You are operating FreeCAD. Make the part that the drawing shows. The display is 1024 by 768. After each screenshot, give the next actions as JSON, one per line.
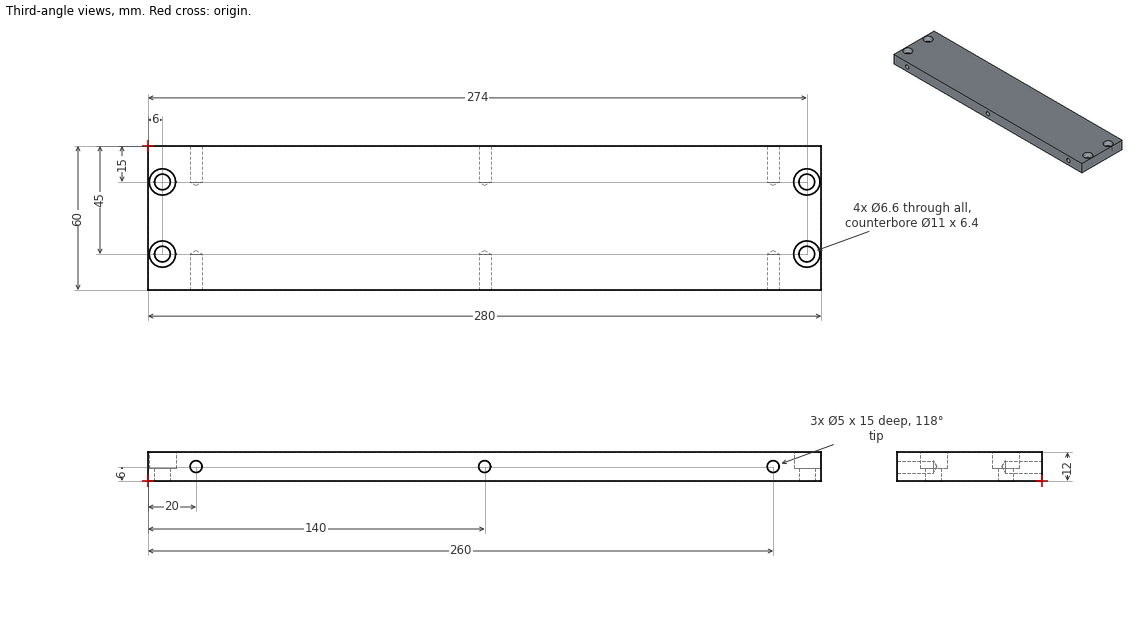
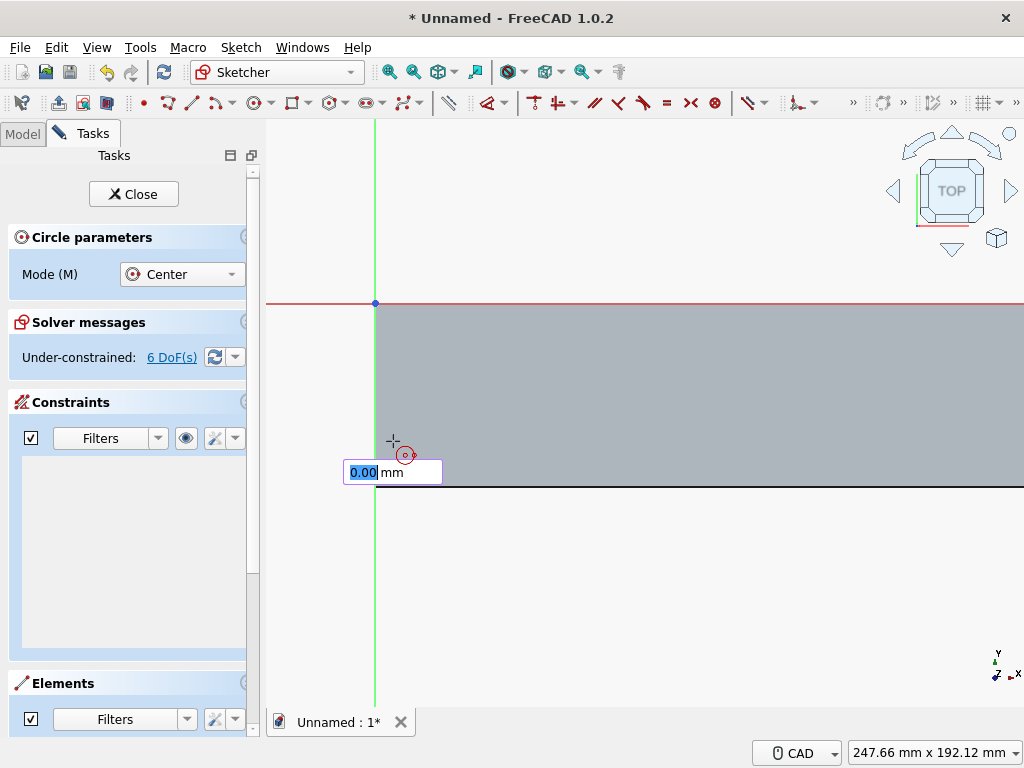
{"action": "scroll", "coordinate": [401, 434], "scroll_direction": "up", "scroll_amount": 3}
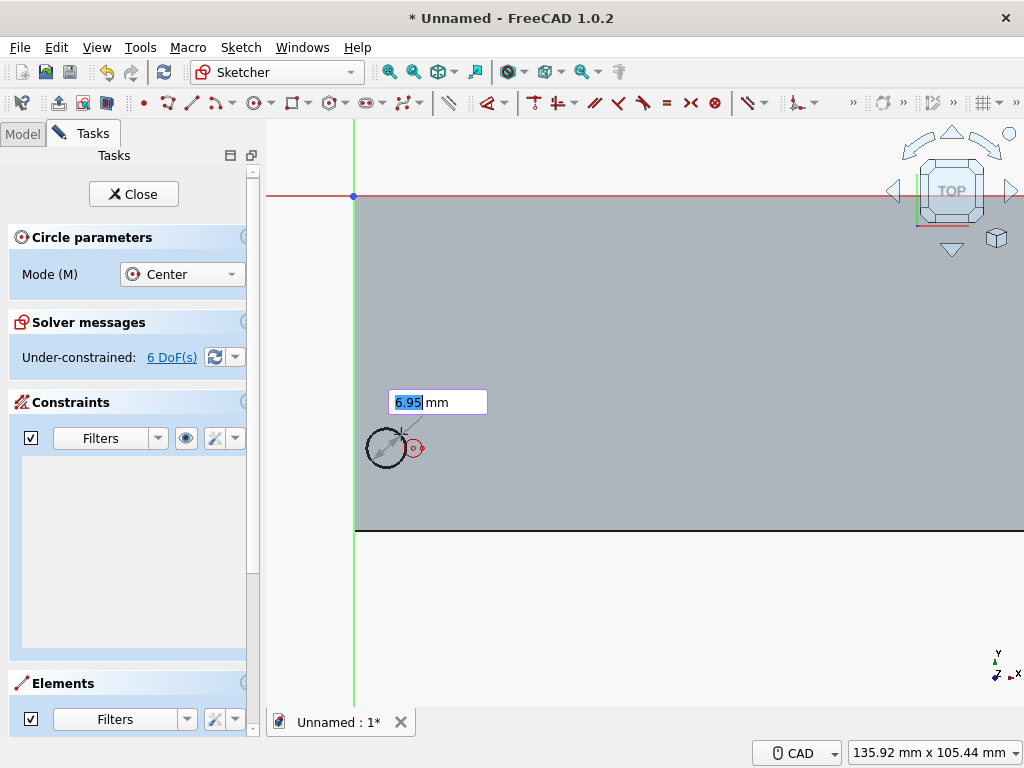
{"action": "left_click", "coordinate": [400, 434]}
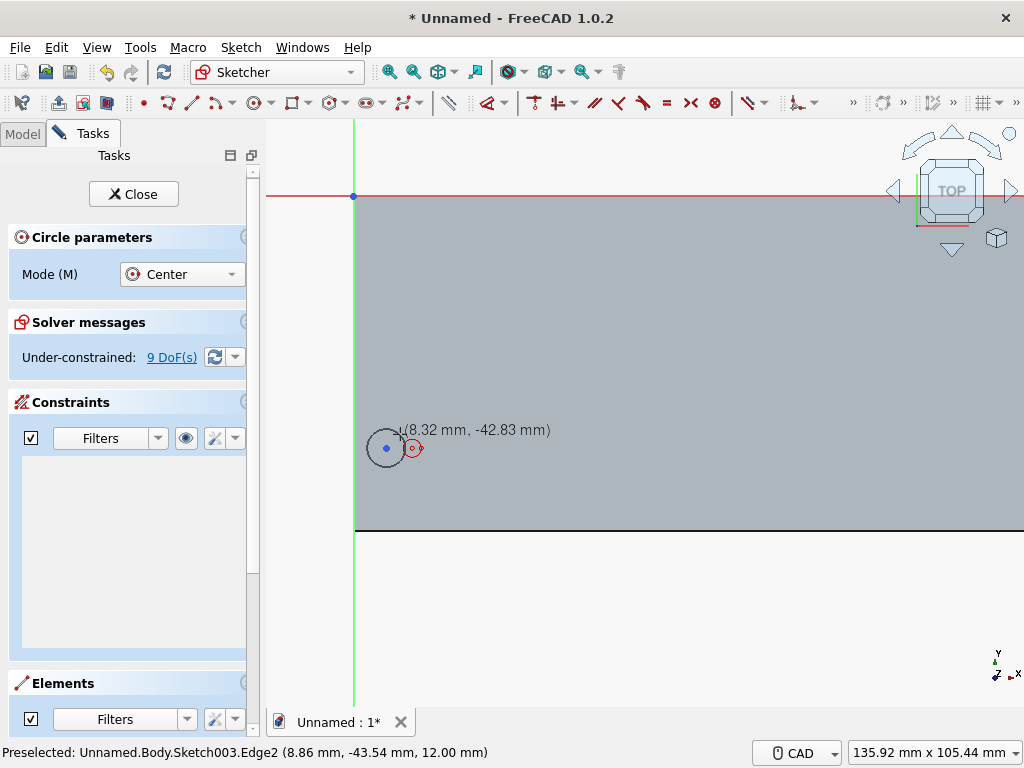
{"action": "scroll", "coordinate": [387, 280], "scroll_direction": "up", "scroll_amount": 2}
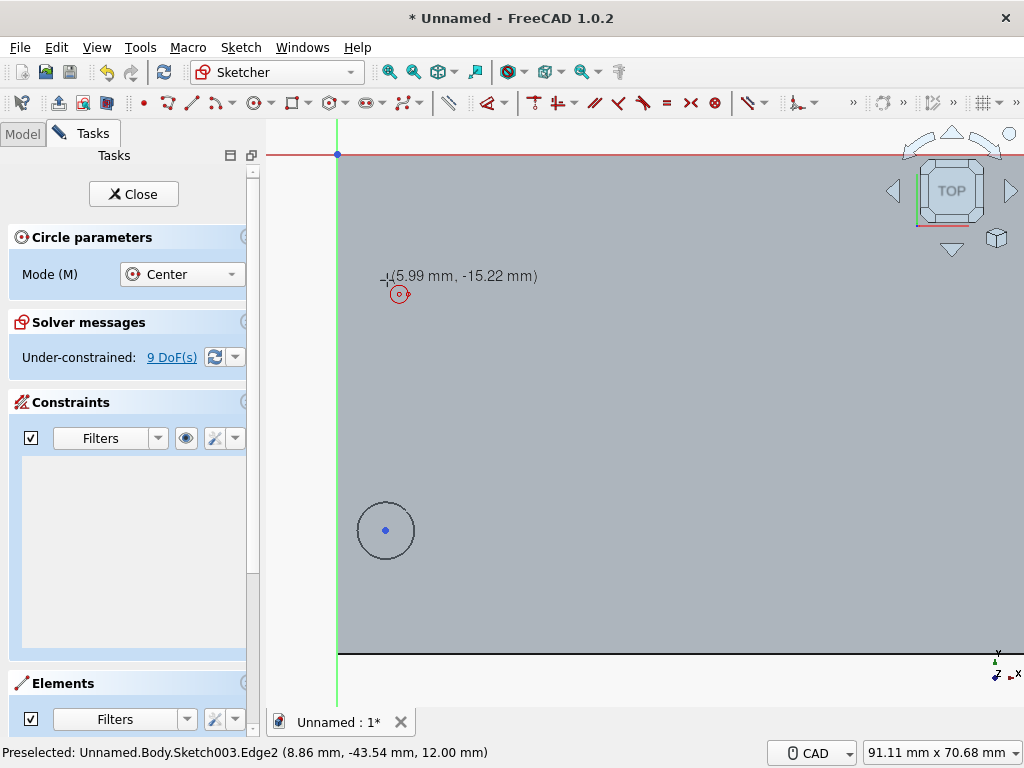
{"action": "scroll", "coordinate": [395, 424], "scroll_direction": "down", "scroll_amount": 9}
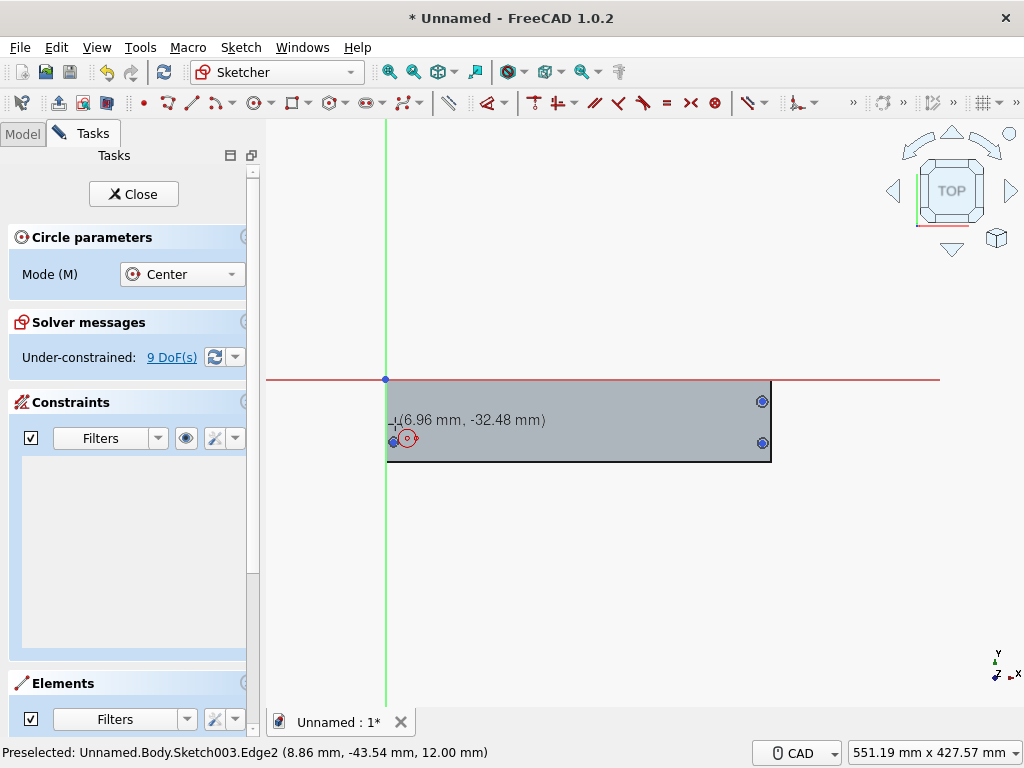
{"action": "scroll", "coordinate": [394, 401], "scroll_direction": "up", "scroll_amount": 4}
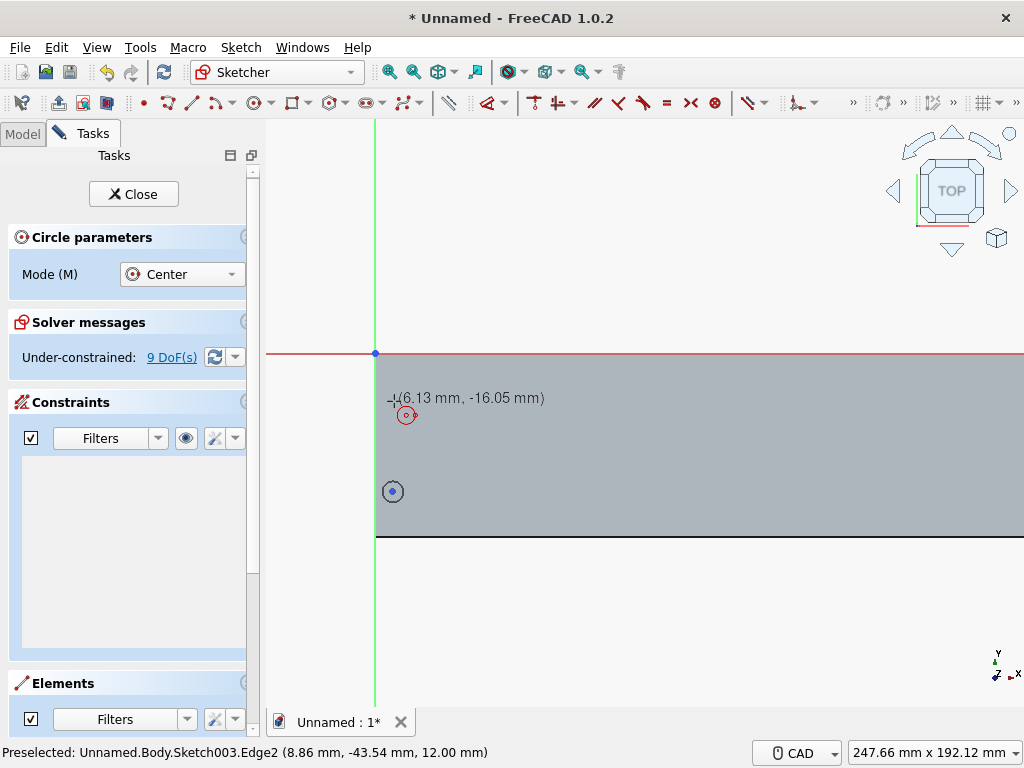
{"action": "left_click", "coordinate": [393, 399]}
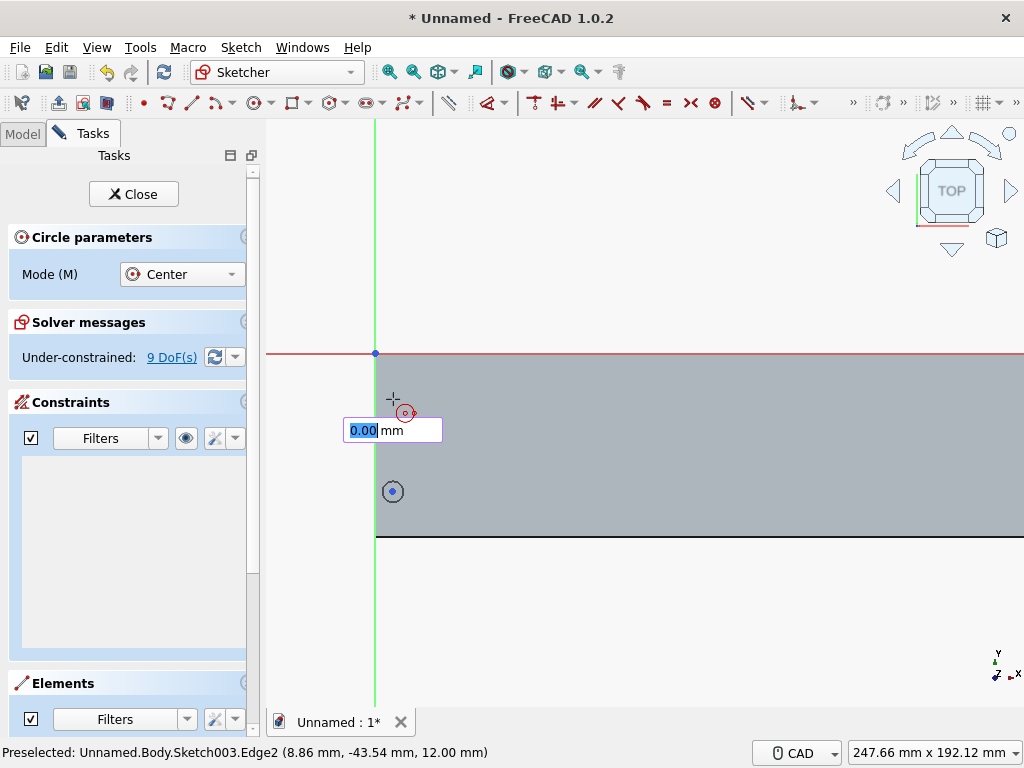
{"action": "scroll", "coordinate": [401, 392], "scroll_direction": "up", "scroll_amount": 3}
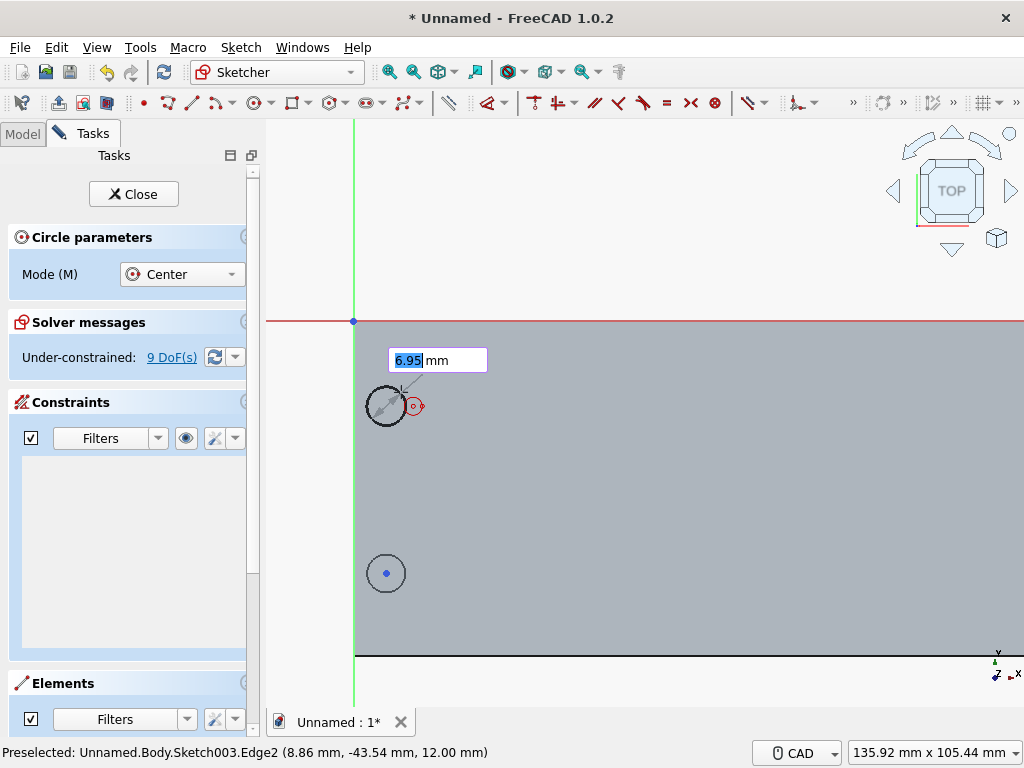
{"action": "left_click", "coordinate": [400, 392]}
{"action": "key", "text": "Escape"}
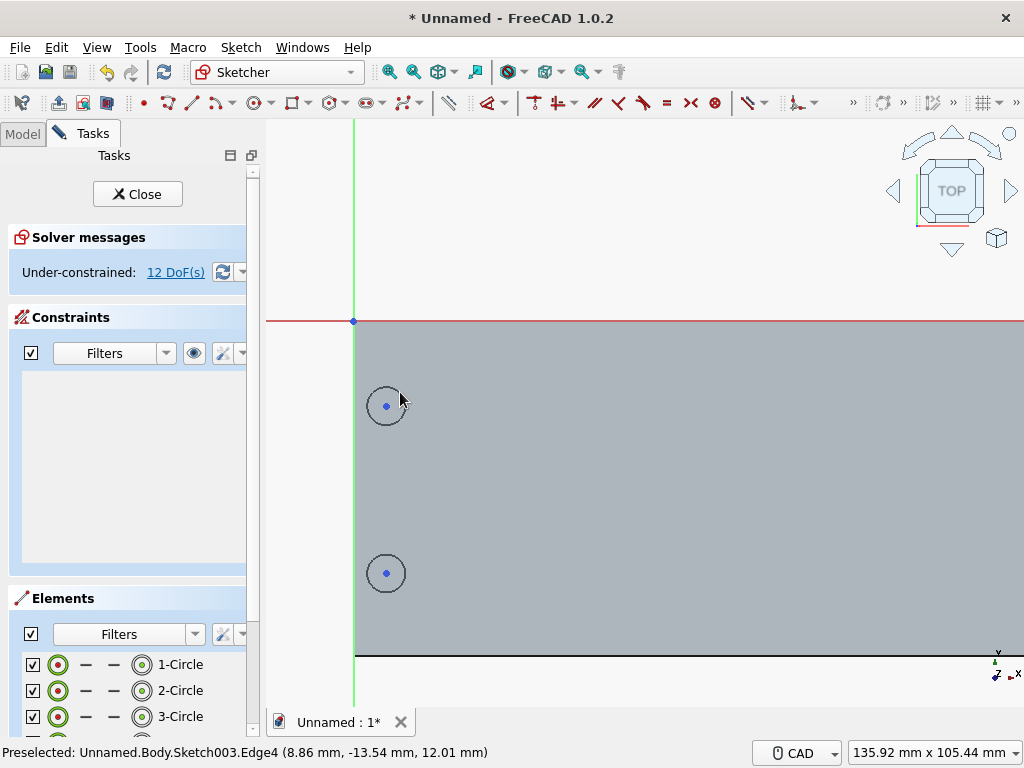
{"action": "scroll", "coordinate": [396, 399], "scroll_direction": "down", "scroll_amount": 7}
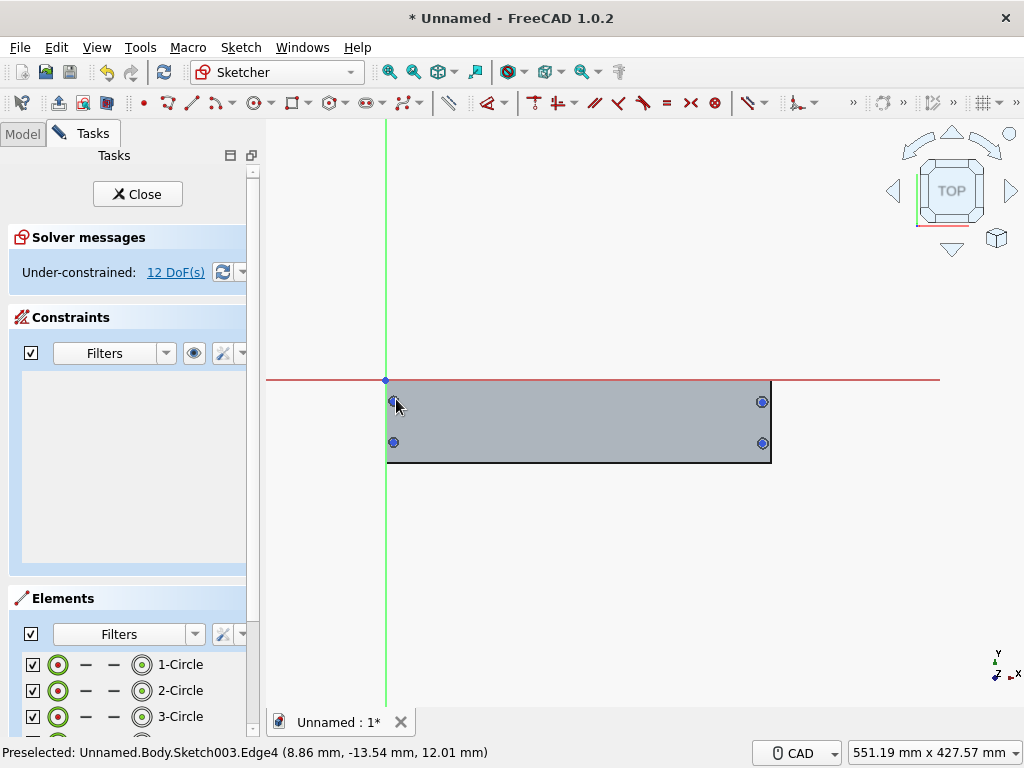
{"action": "scroll", "coordinate": [766, 440], "scroll_direction": "up", "scroll_amount": 5}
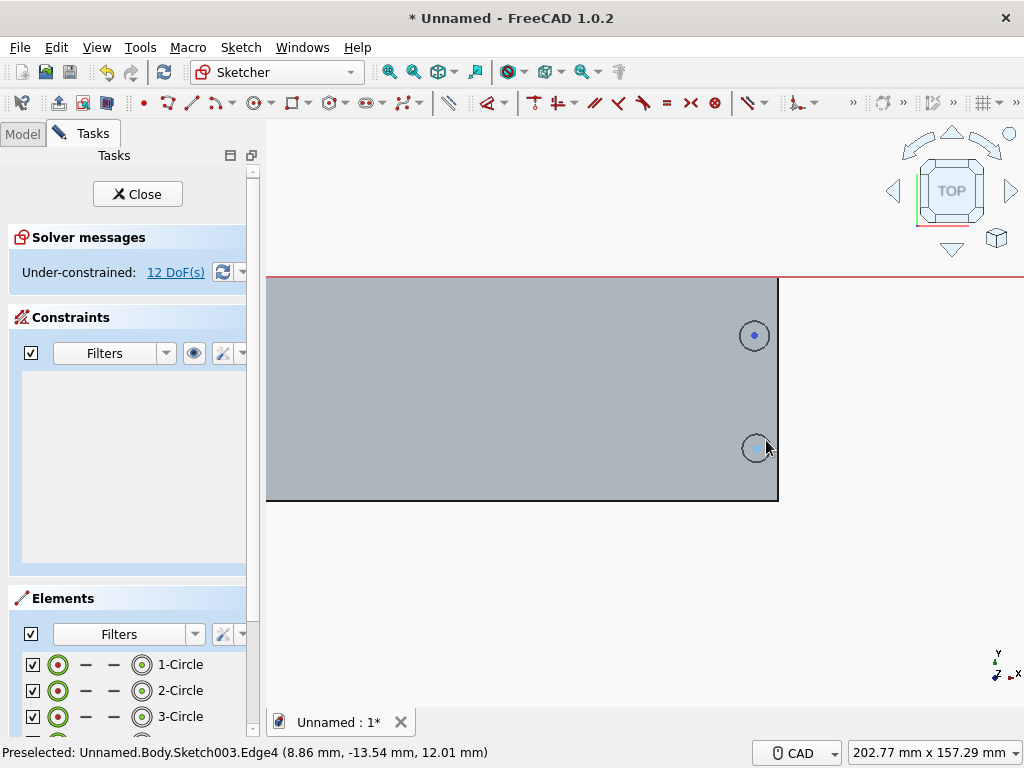
{"action": "left_click", "coordinate": [766, 438]}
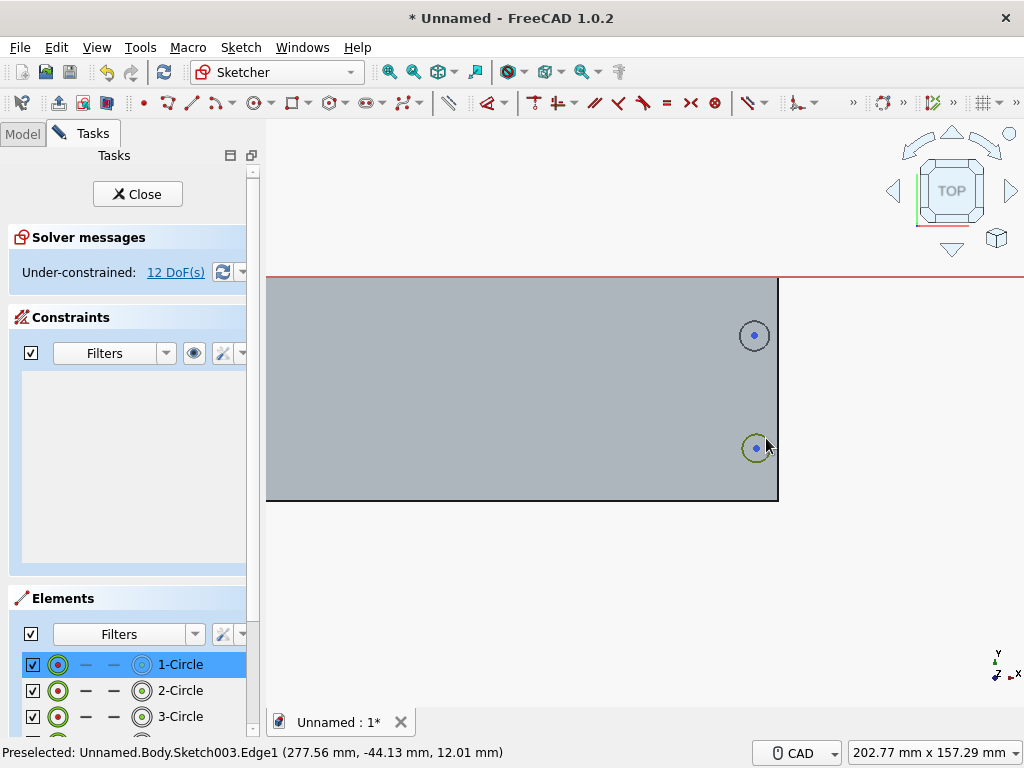
{"action": "left_click", "coordinate": [765, 326]}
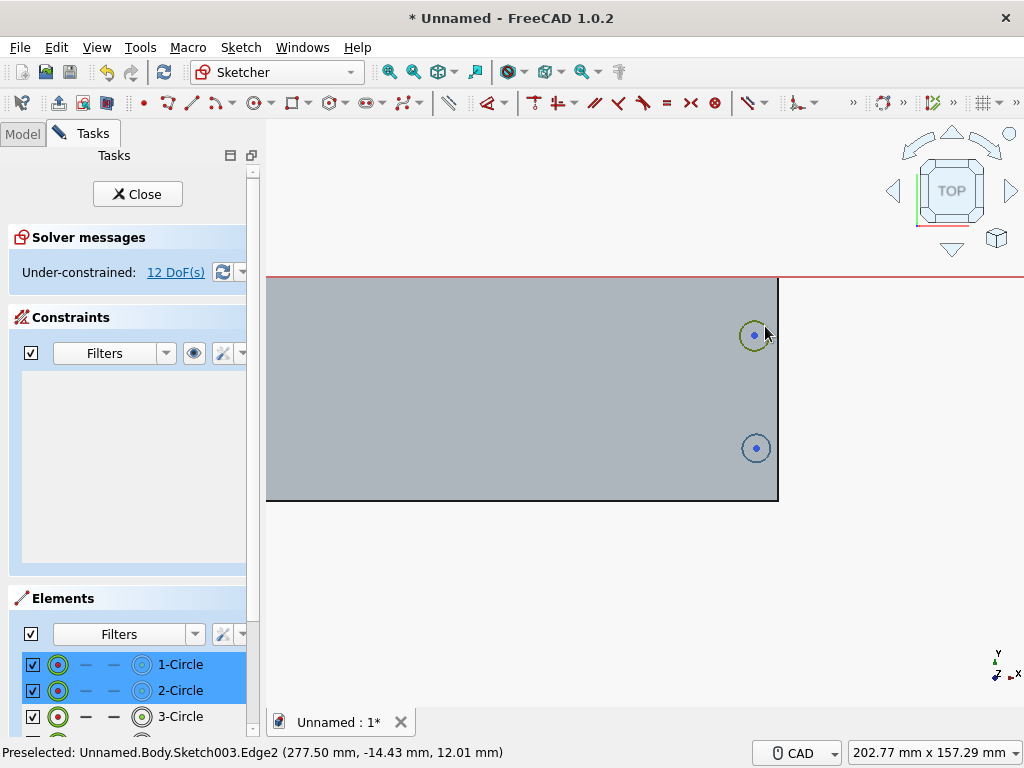
{"action": "scroll", "coordinate": [767, 440], "scroll_direction": "down", "scroll_amount": 5}